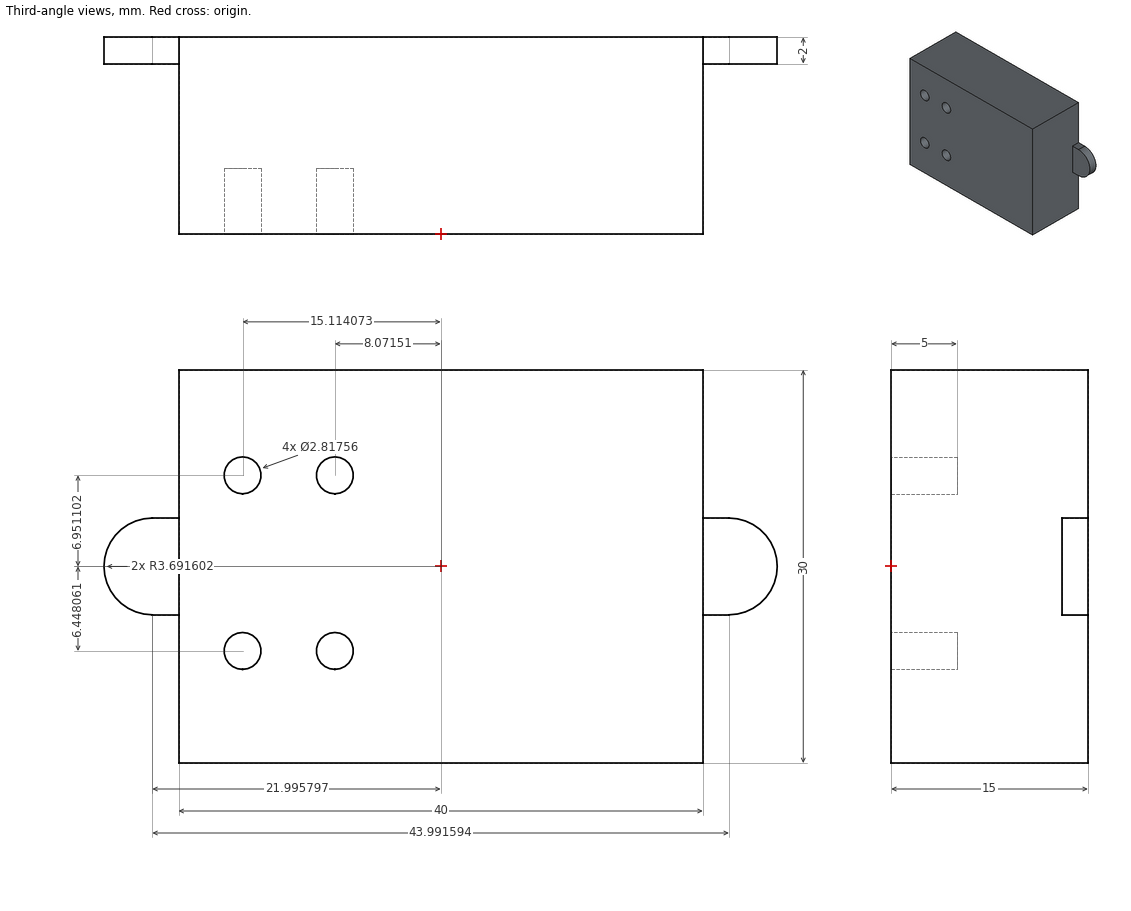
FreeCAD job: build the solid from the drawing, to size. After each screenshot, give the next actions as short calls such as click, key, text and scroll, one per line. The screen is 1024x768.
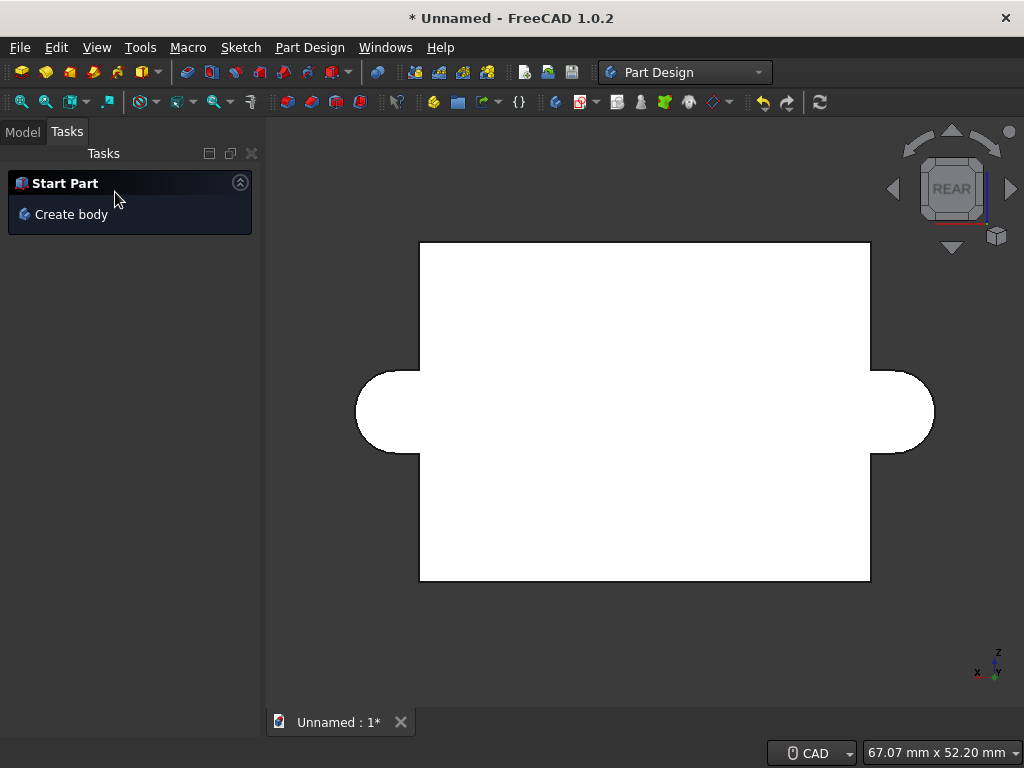
key(0)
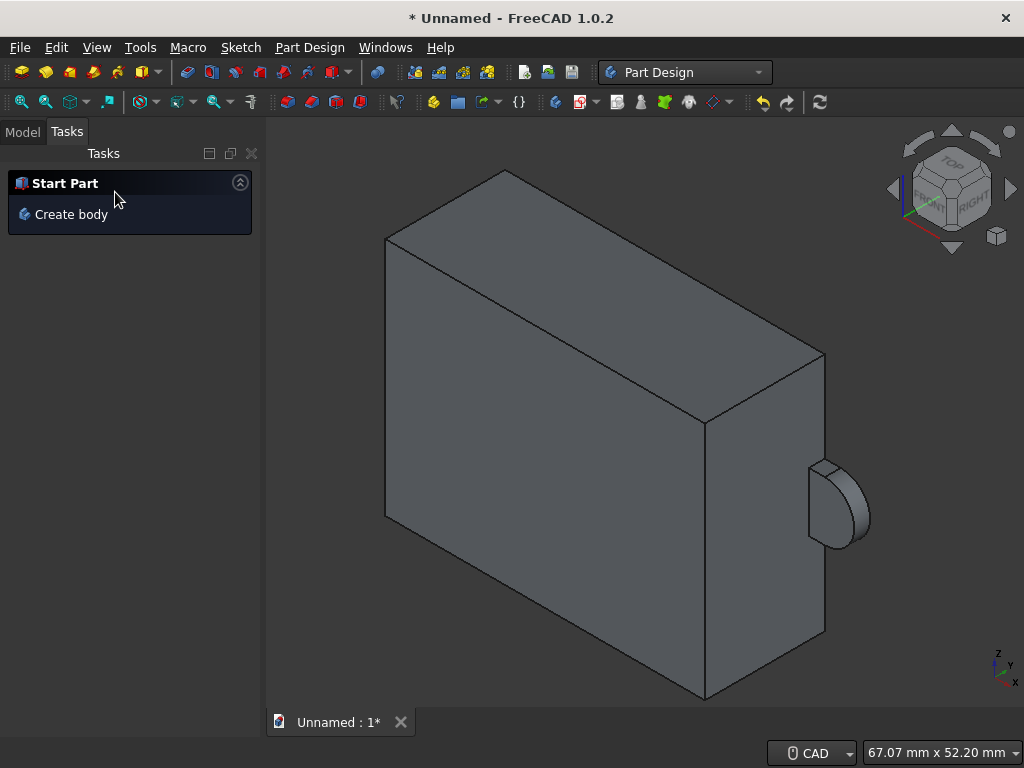
click(22, 102)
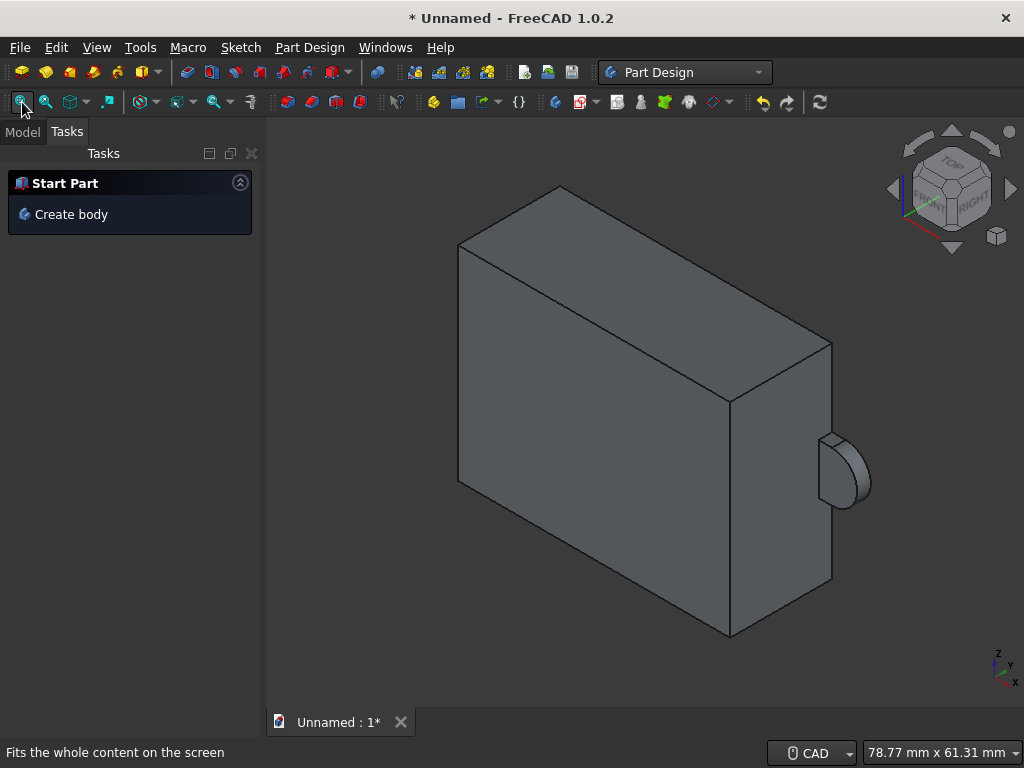
click(594, 440)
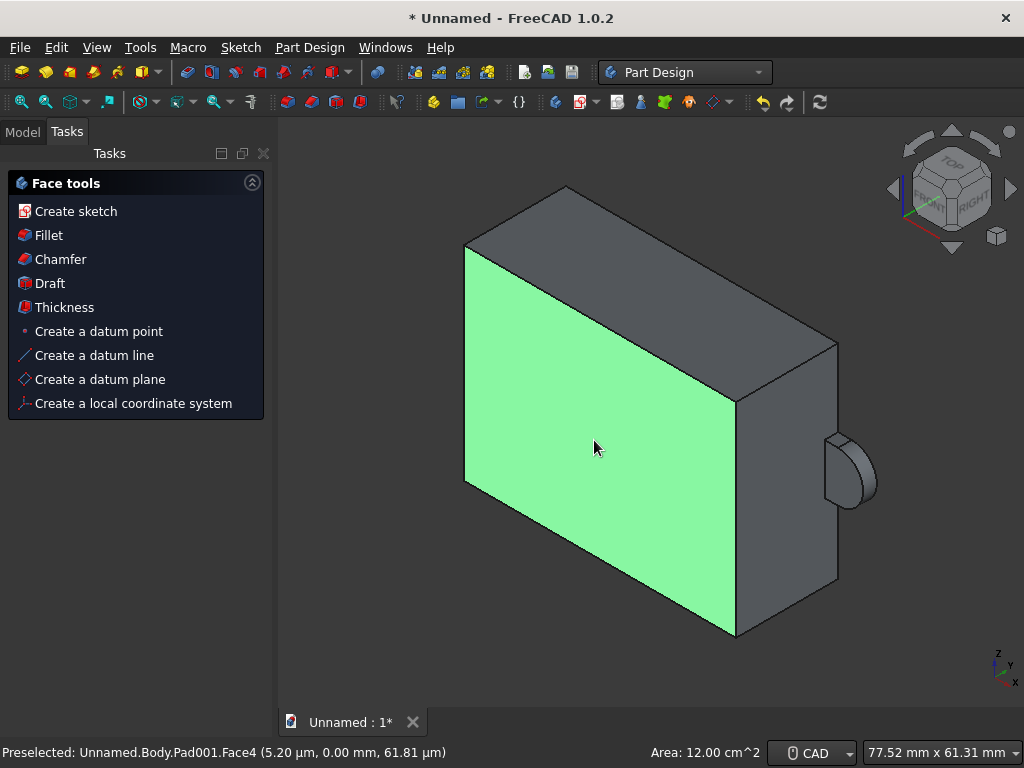
click(580, 102)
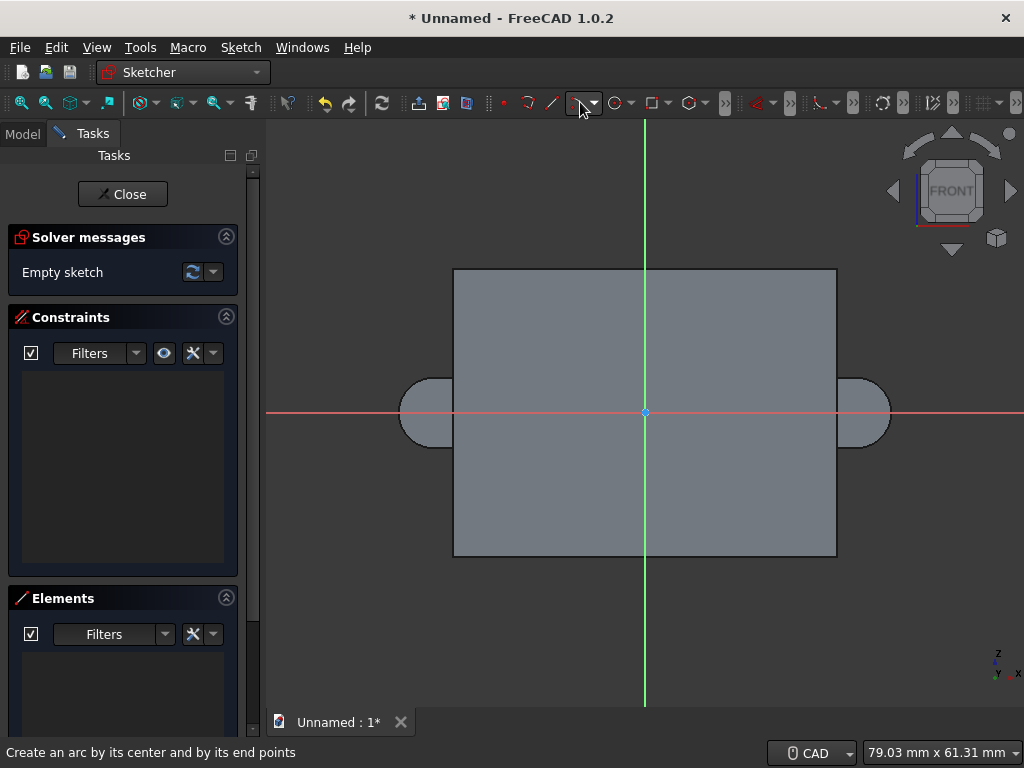
scroll(557, 409, up, 4)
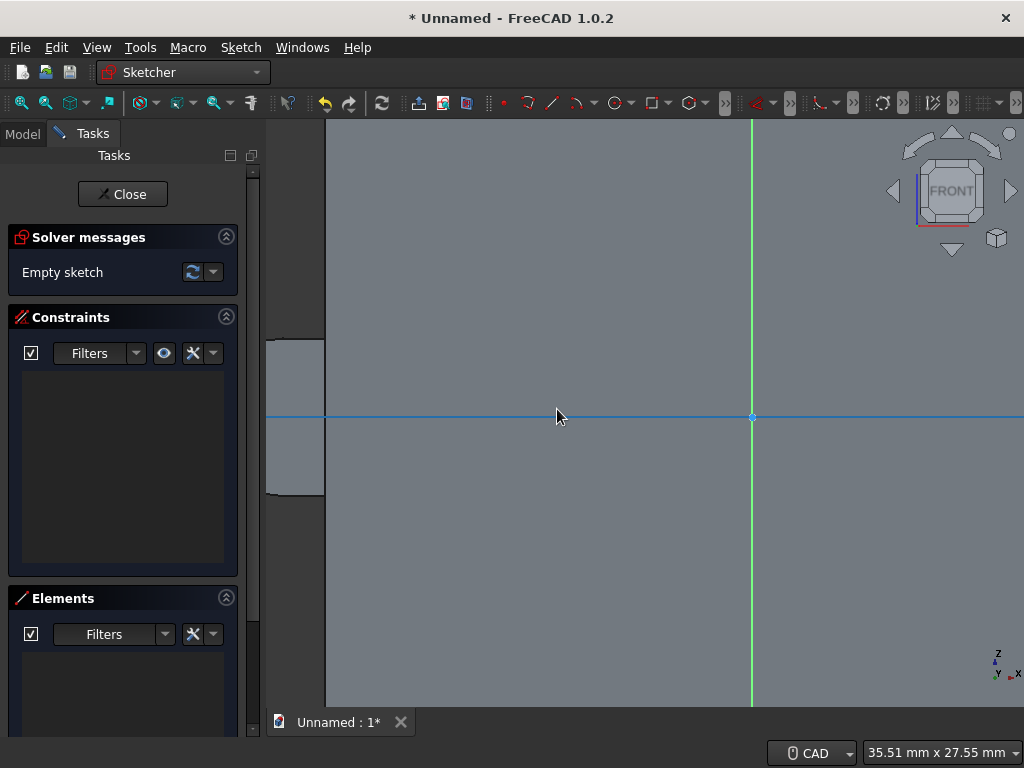
click(616, 104)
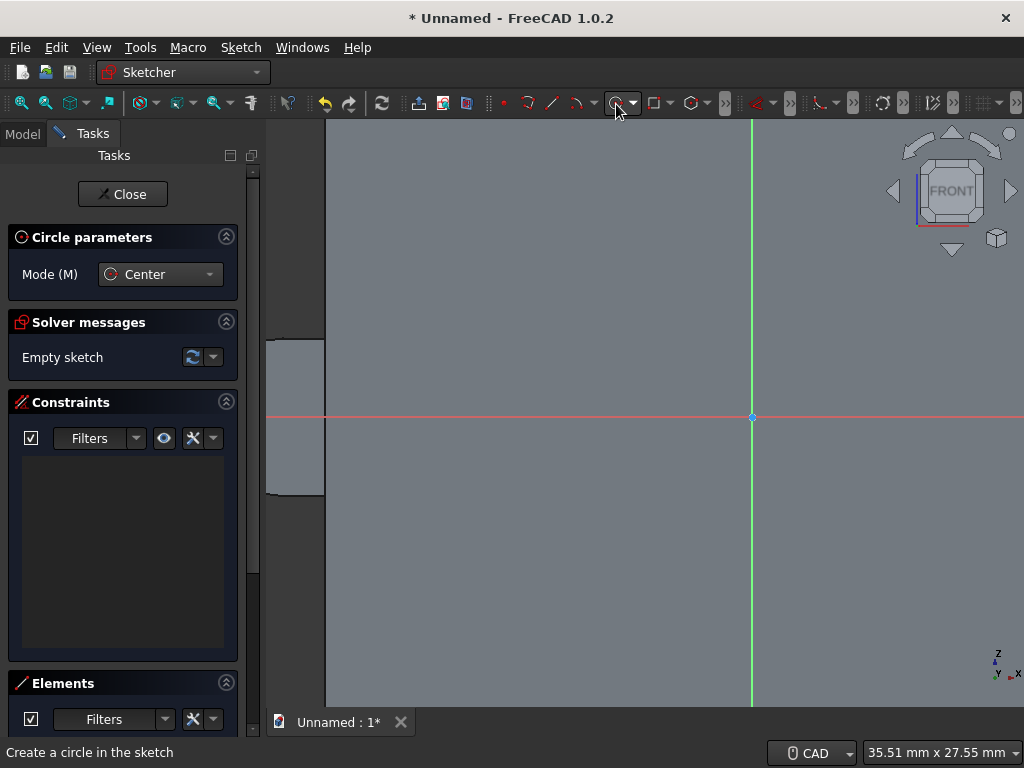
click(430, 269)
click(451, 248)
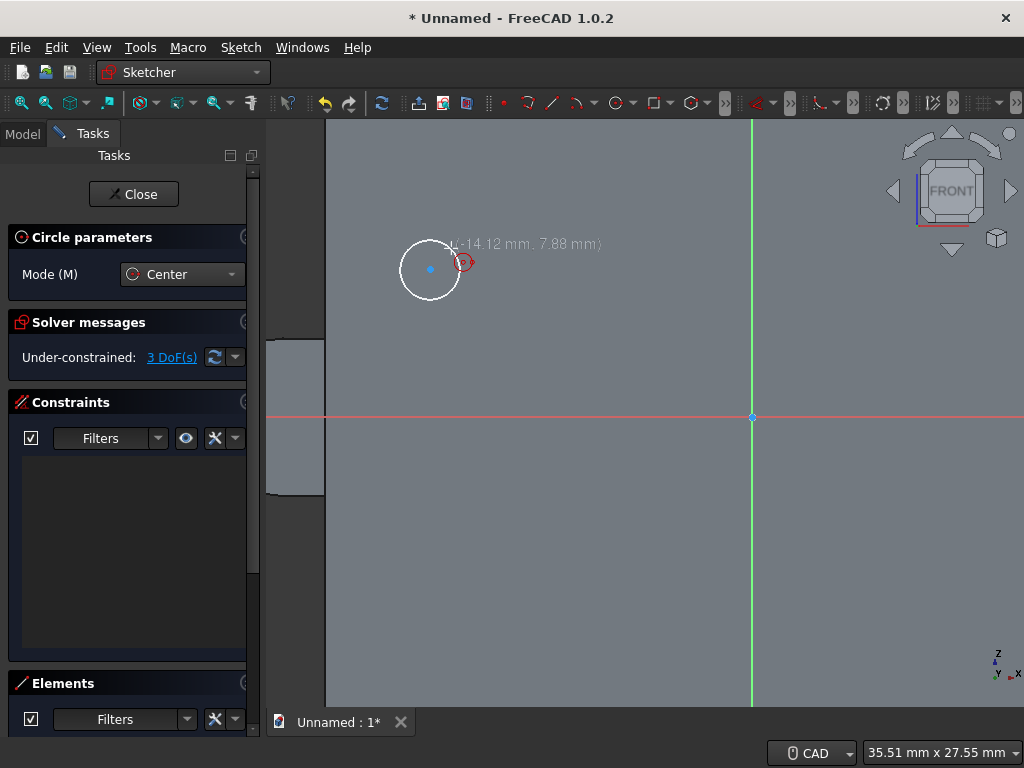
click(580, 269)
click(601, 248)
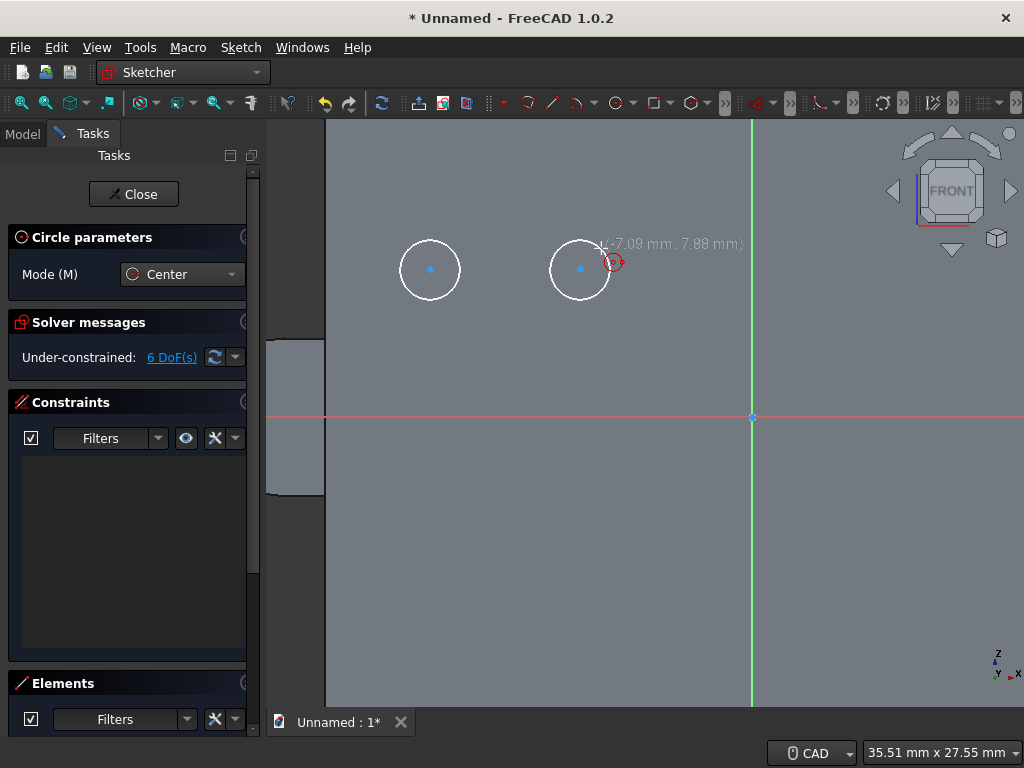
click(430, 555)
click(451, 534)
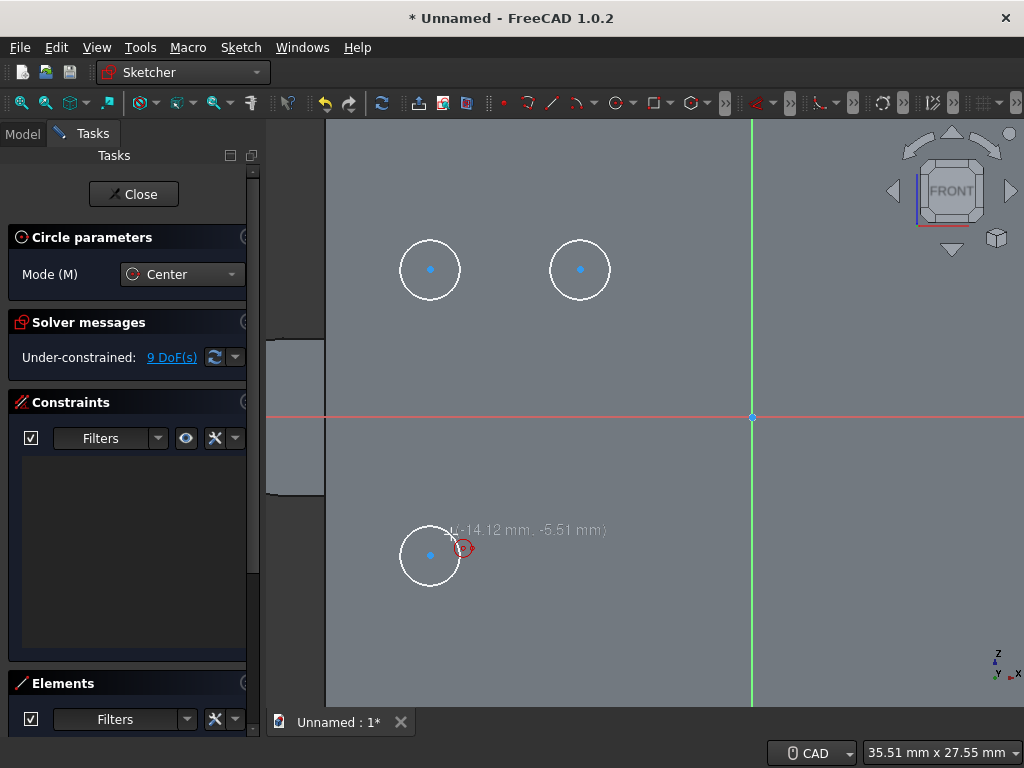
click(580, 555)
click(601, 534)
key(Escape)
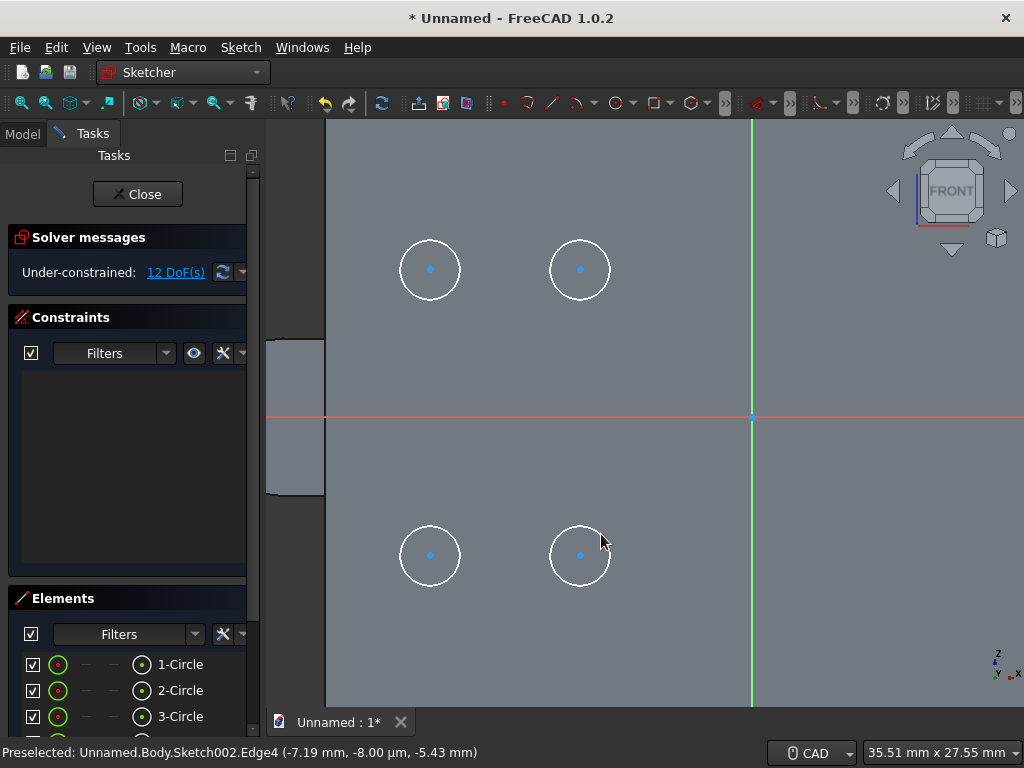
click(451, 249)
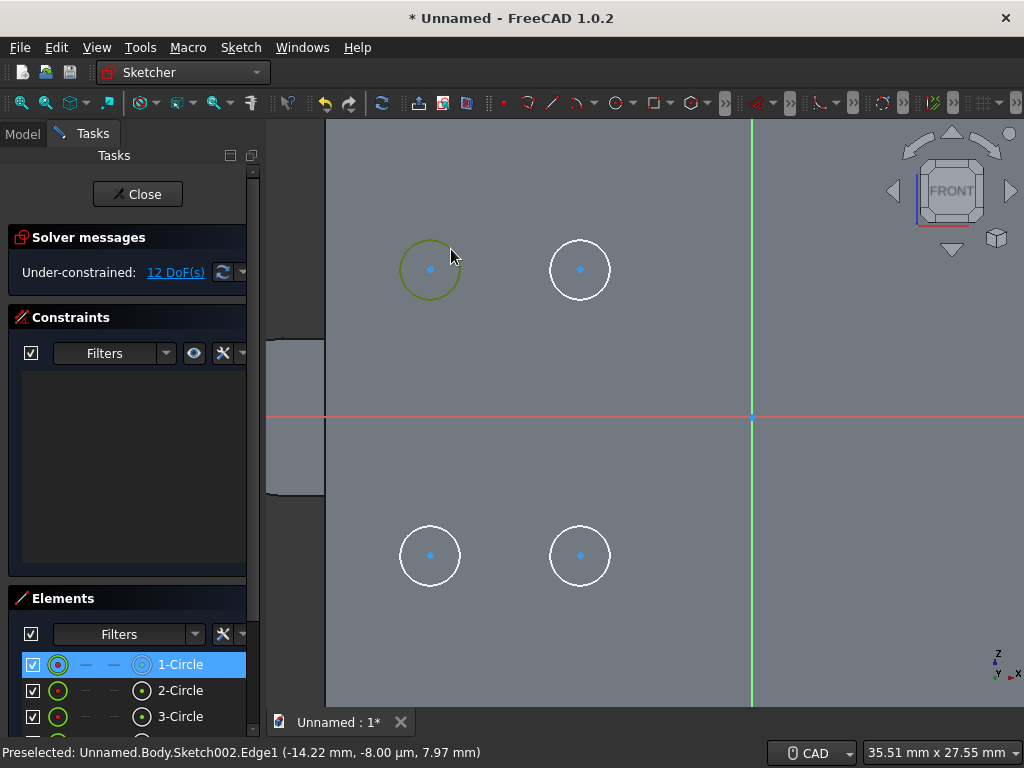
click(601, 249)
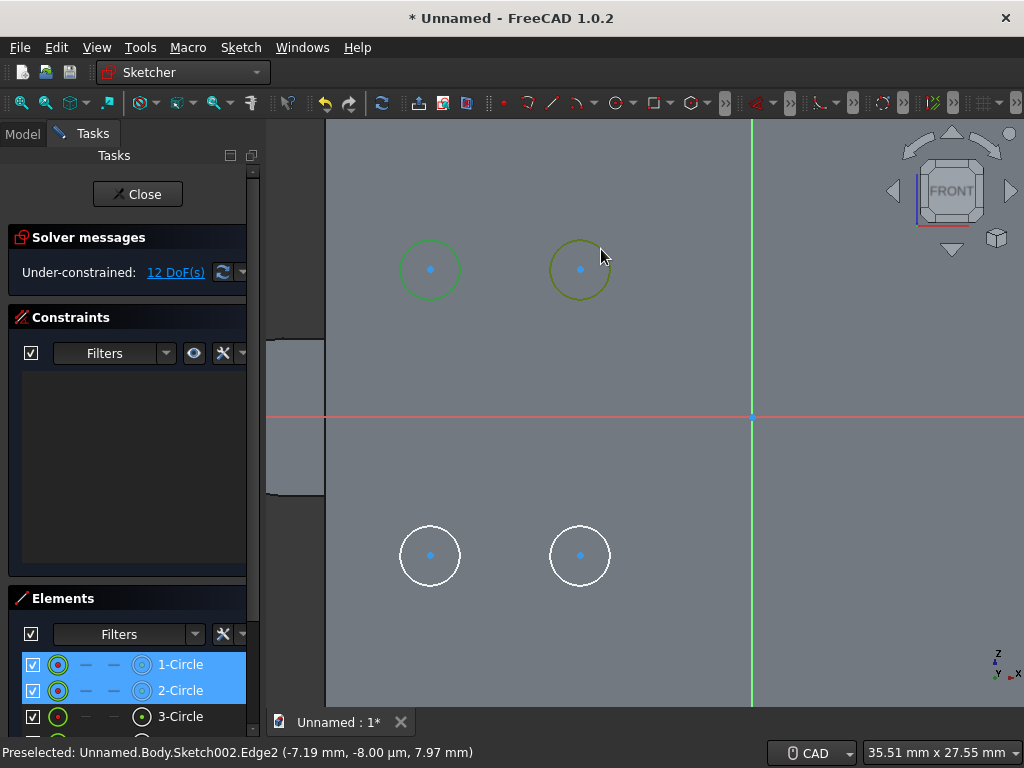
click(451, 535)